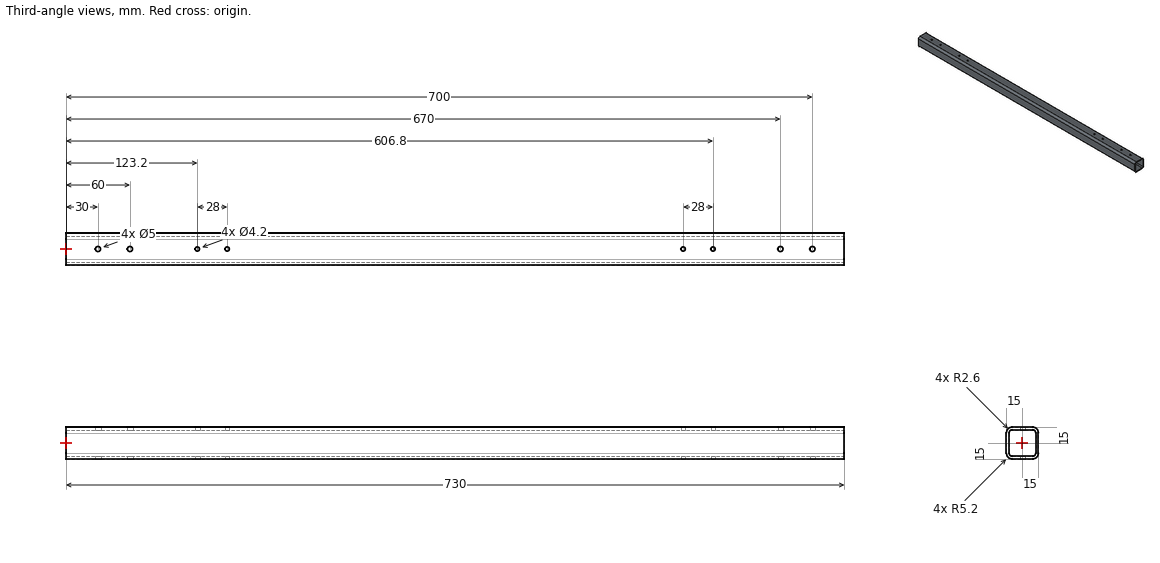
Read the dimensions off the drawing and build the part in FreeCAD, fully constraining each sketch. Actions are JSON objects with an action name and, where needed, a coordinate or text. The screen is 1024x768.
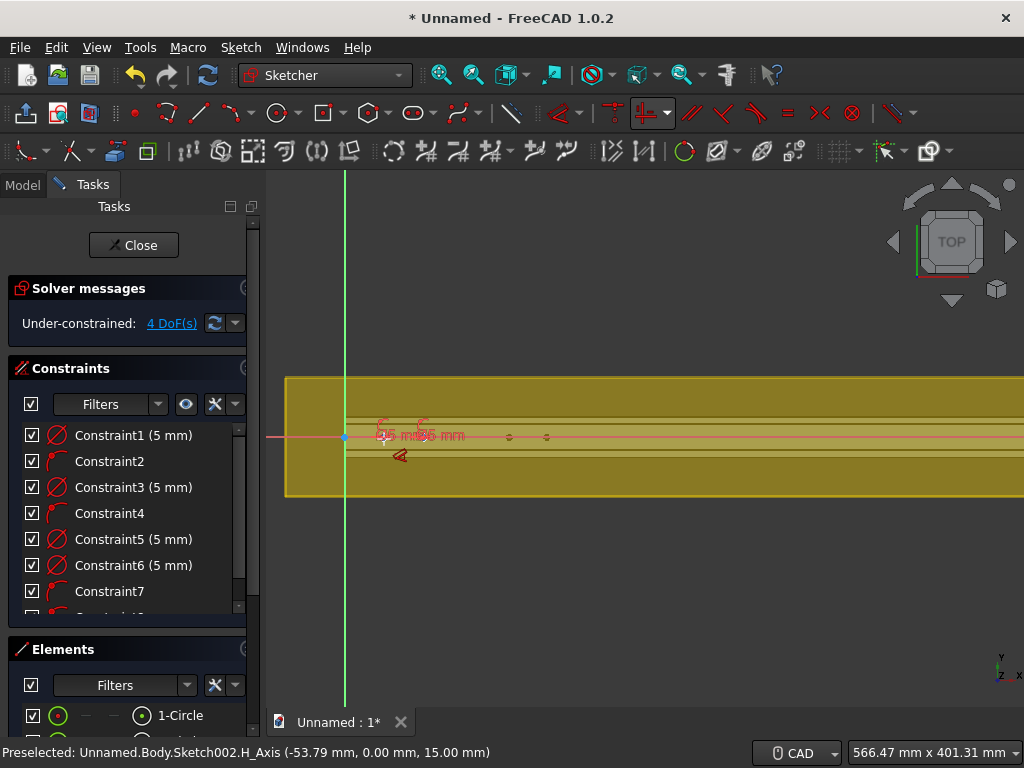
{"action": "left_click", "coordinate": [384, 437]}
{"action": "left_click", "coordinate": [364, 471]}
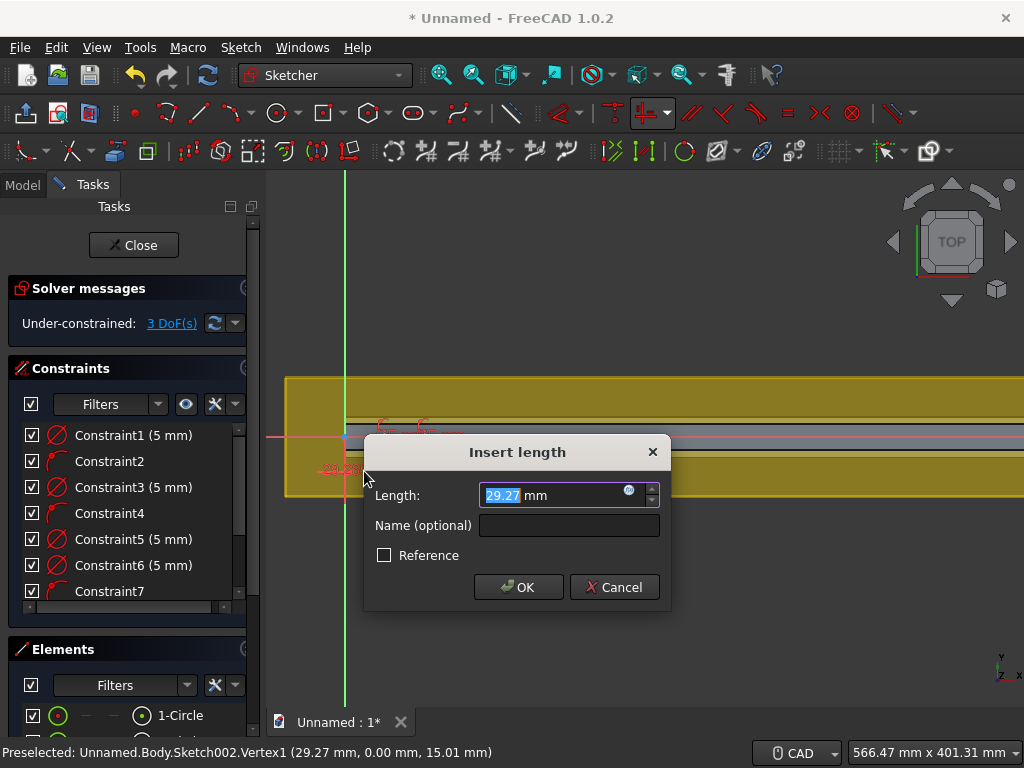
{"action": "type", "text": "30"}
{"action": "key", "text": "Return"}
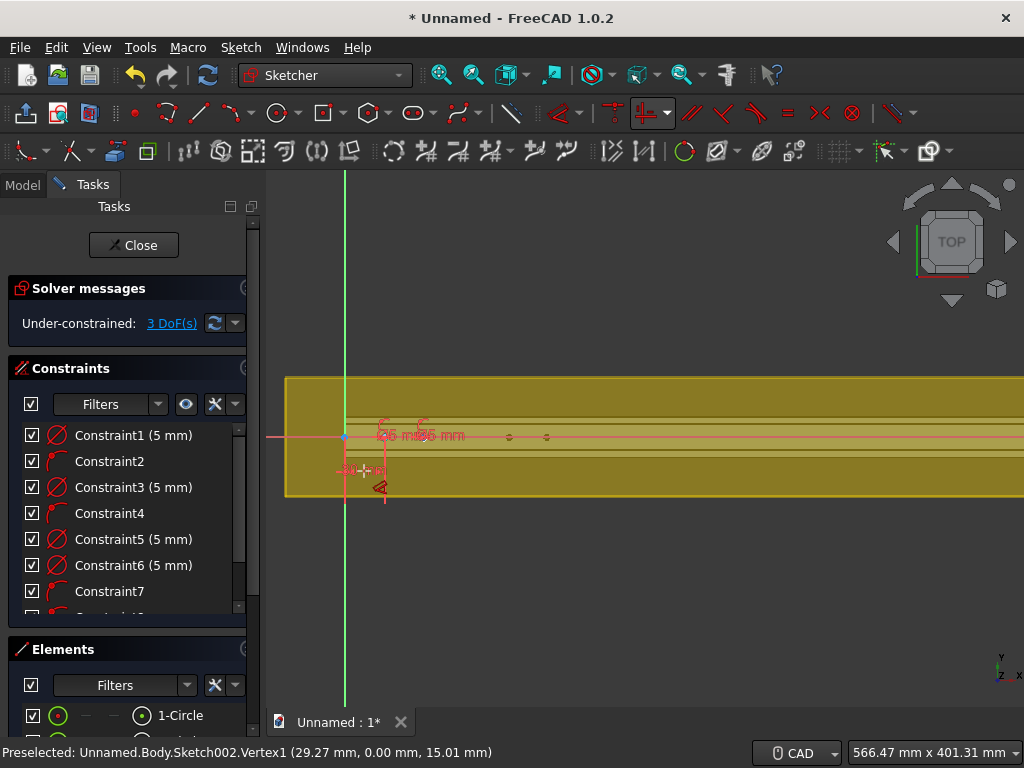
{"action": "left_click", "coordinate": [424, 437]}
{"action": "left_click", "coordinate": [384, 403]}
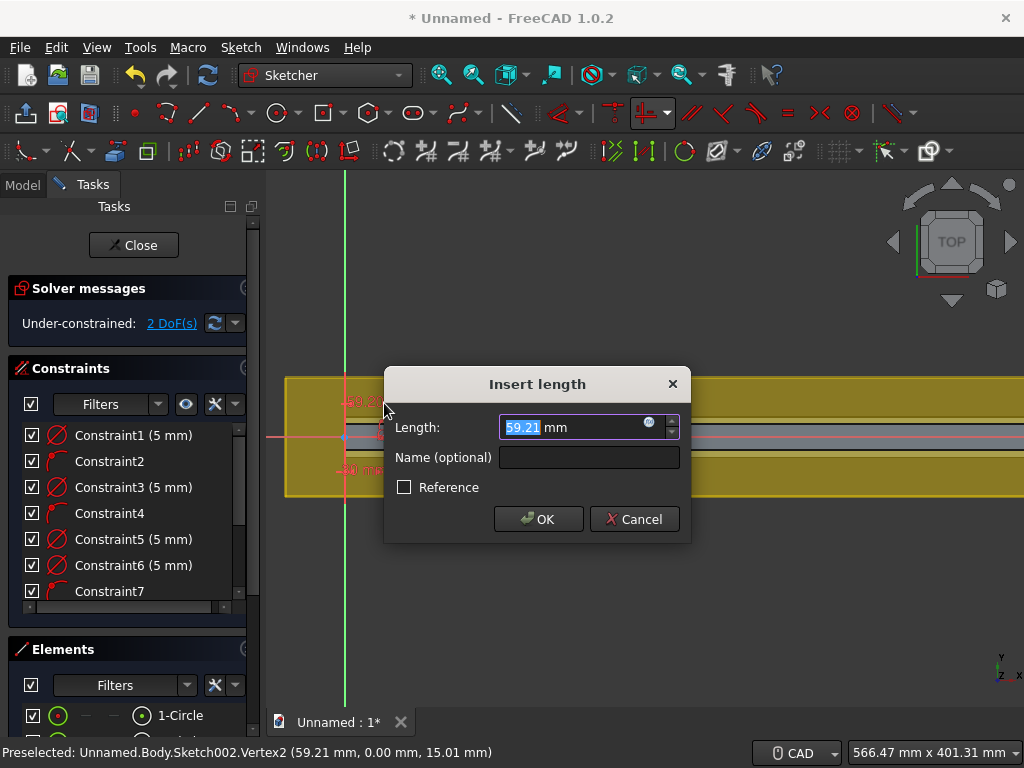
{"action": "type", "text": "60"}
{"action": "key", "text": "Return"}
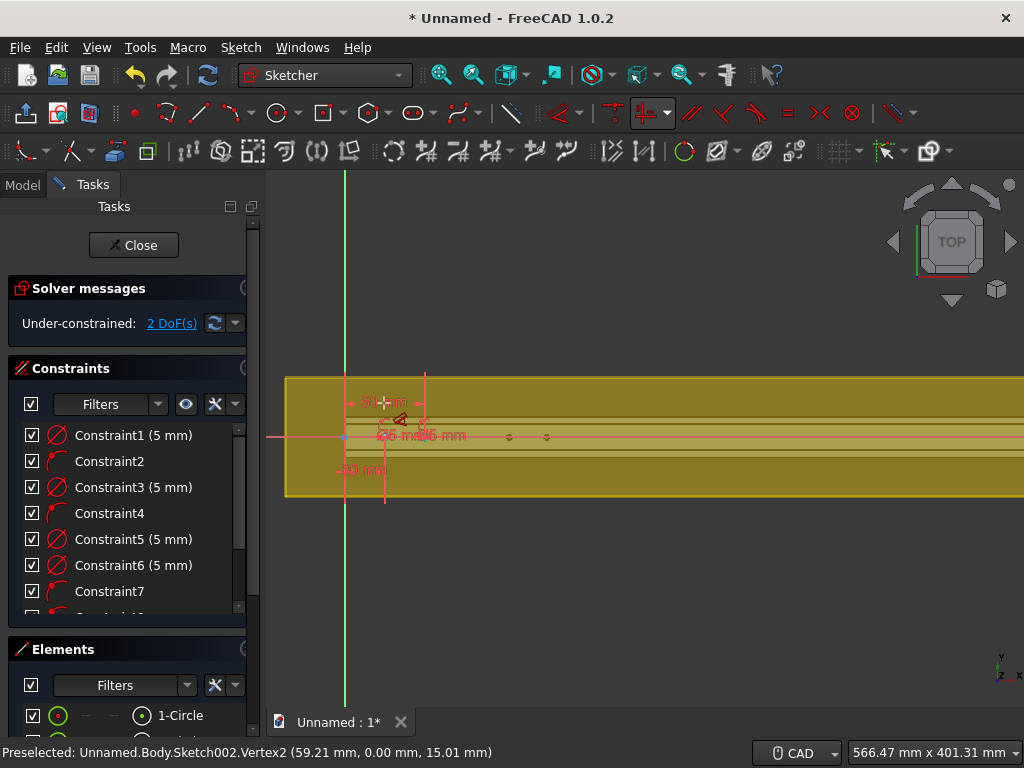
{"action": "scroll", "coordinate": [382, 439], "scroll_direction": "down", "scroll_amount": 4}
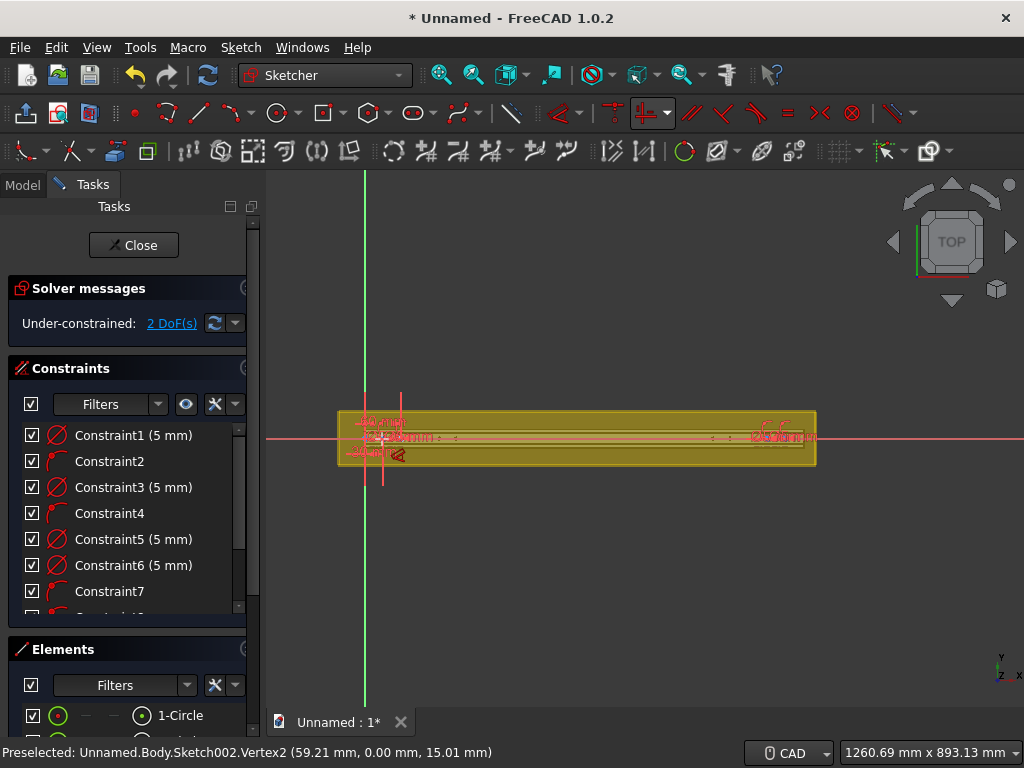
{"action": "left_click", "coordinate": [786, 439]}
{"action": "left_click", "coordinate": [576, 473]}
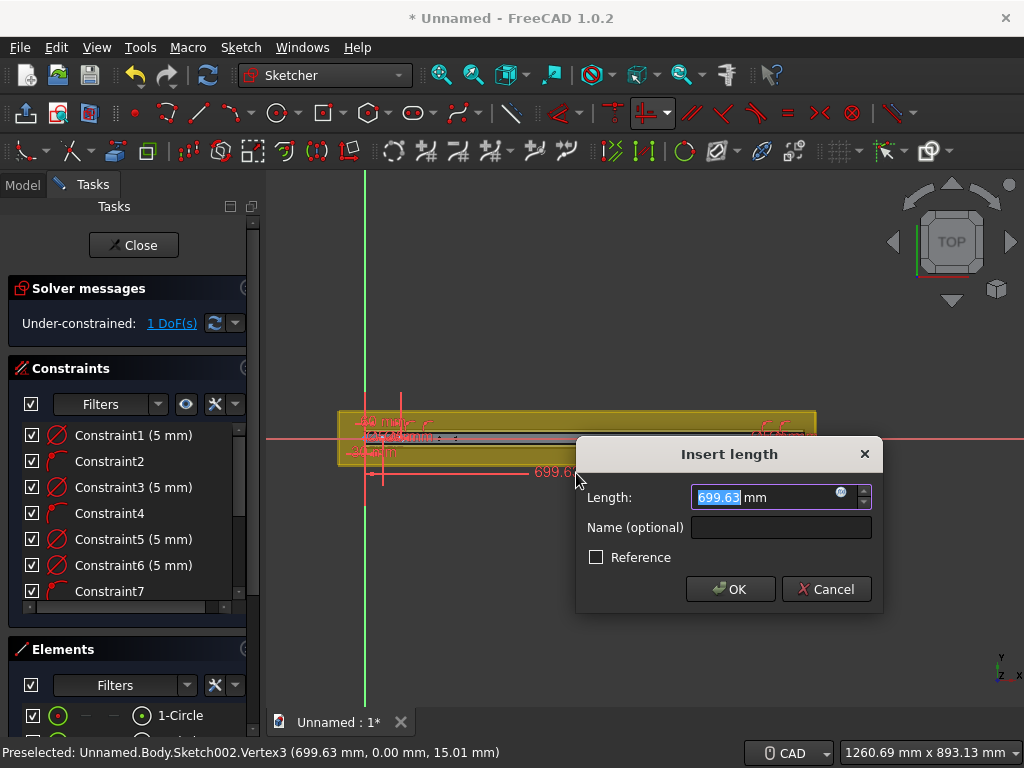
{"action": "type", "text": "700"}
{"action": "key", "text": "Return"}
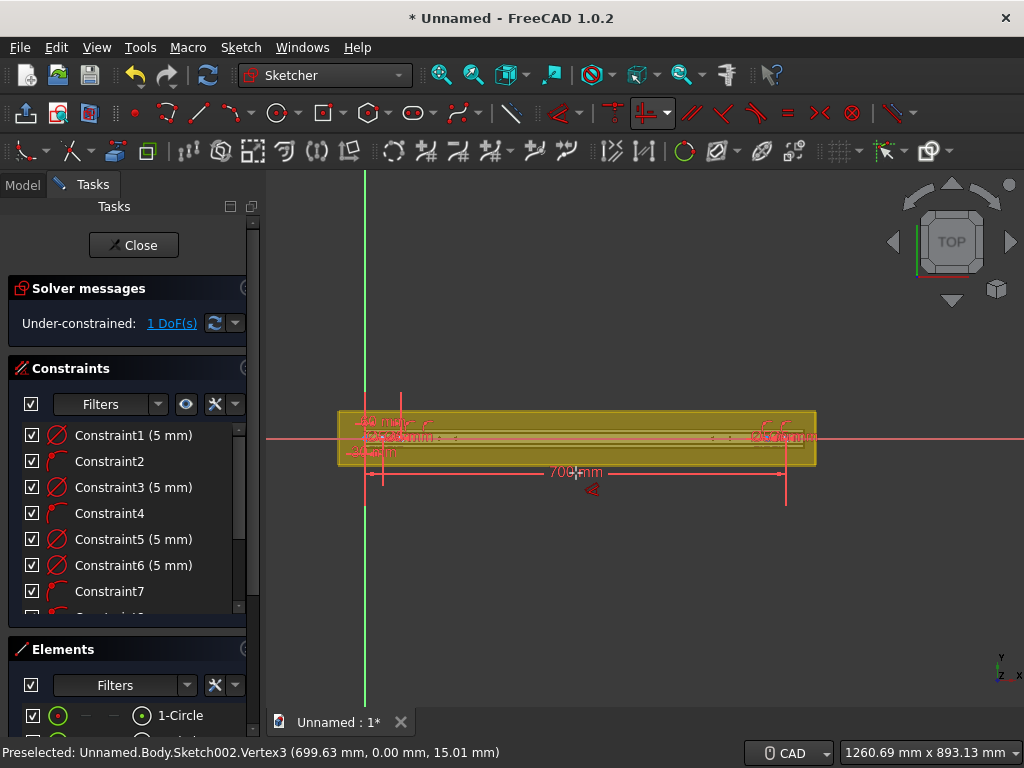
{"action": "left_click", "coordinate": [768, 439]}
{"action": "left_click", "coordinate": [474, 473]}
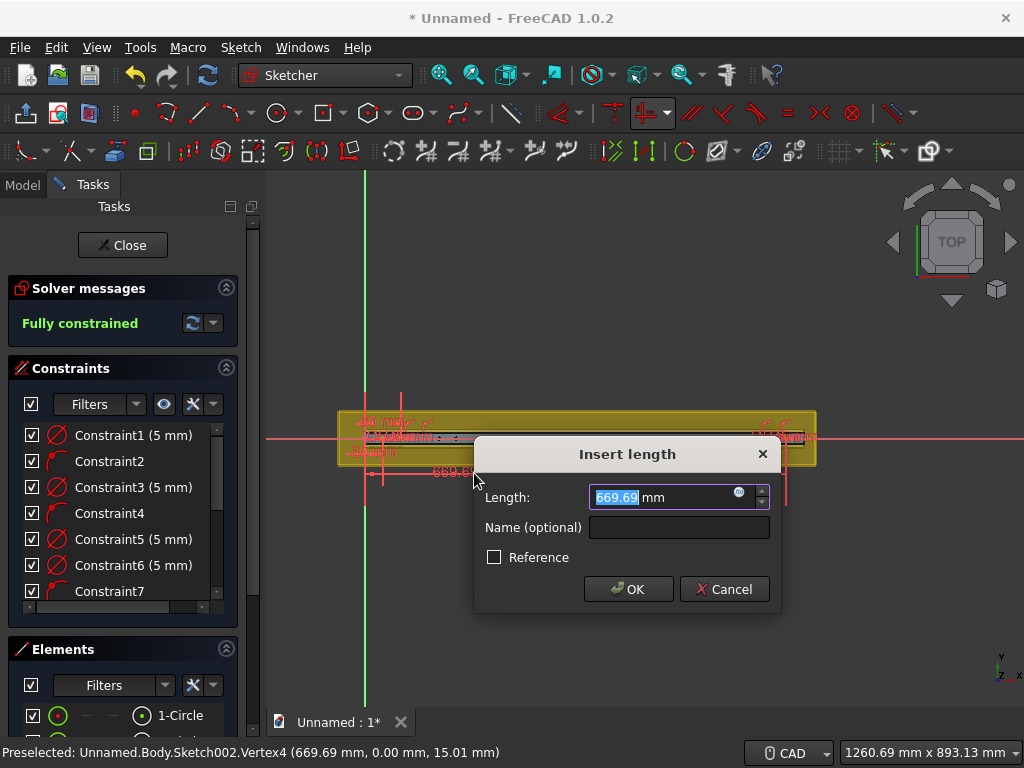
{"action": "type", "text": "670"}
{"action": "key", "text": "Return"}
{"action": "key", "text": "Escape"}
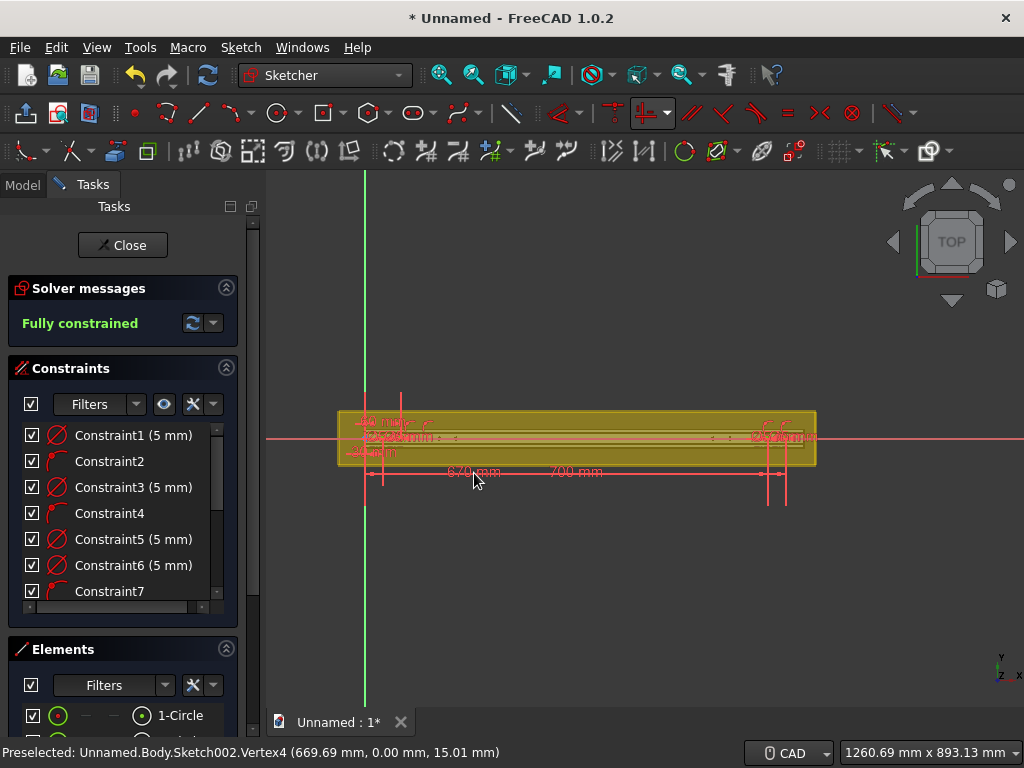
{"action": "left_click", "coordinate": [123, 245]}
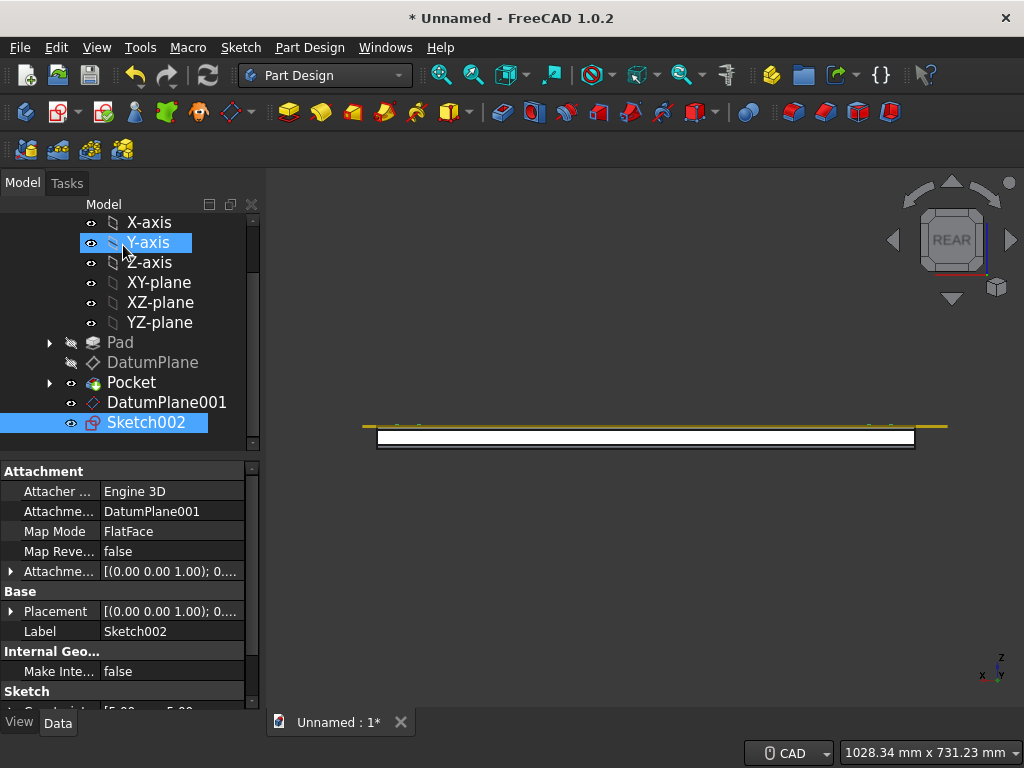
{"action": "left_click", "coordinate": [504, 112]}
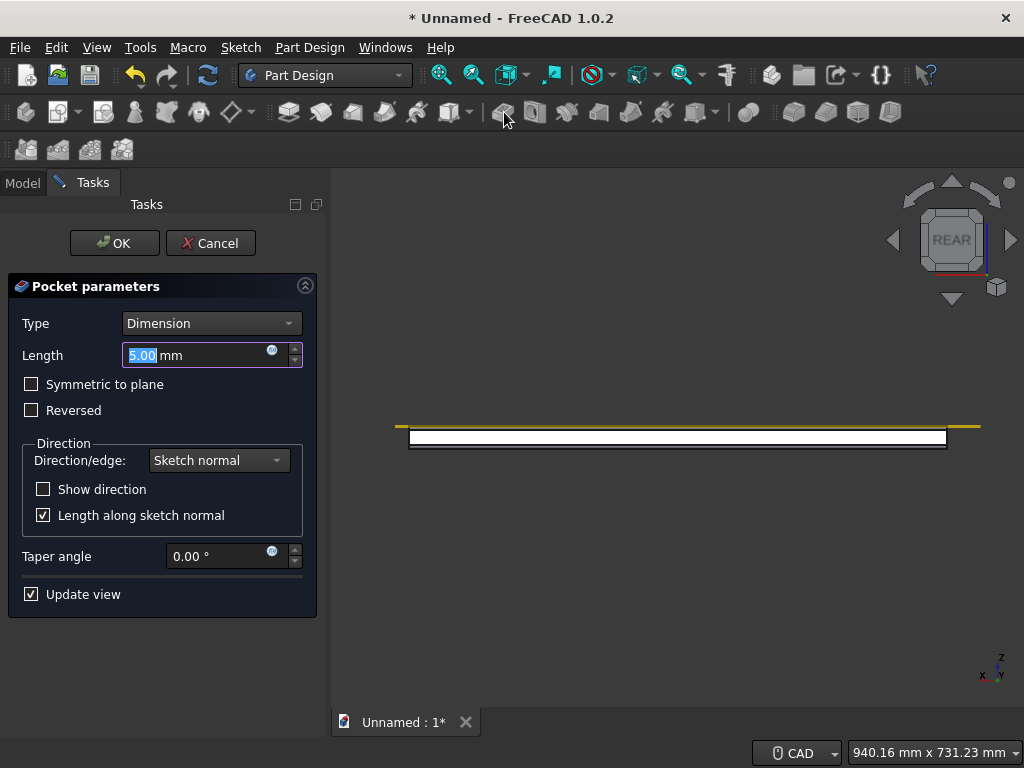
{"action": "left_click", "coordinate": [212, 324]}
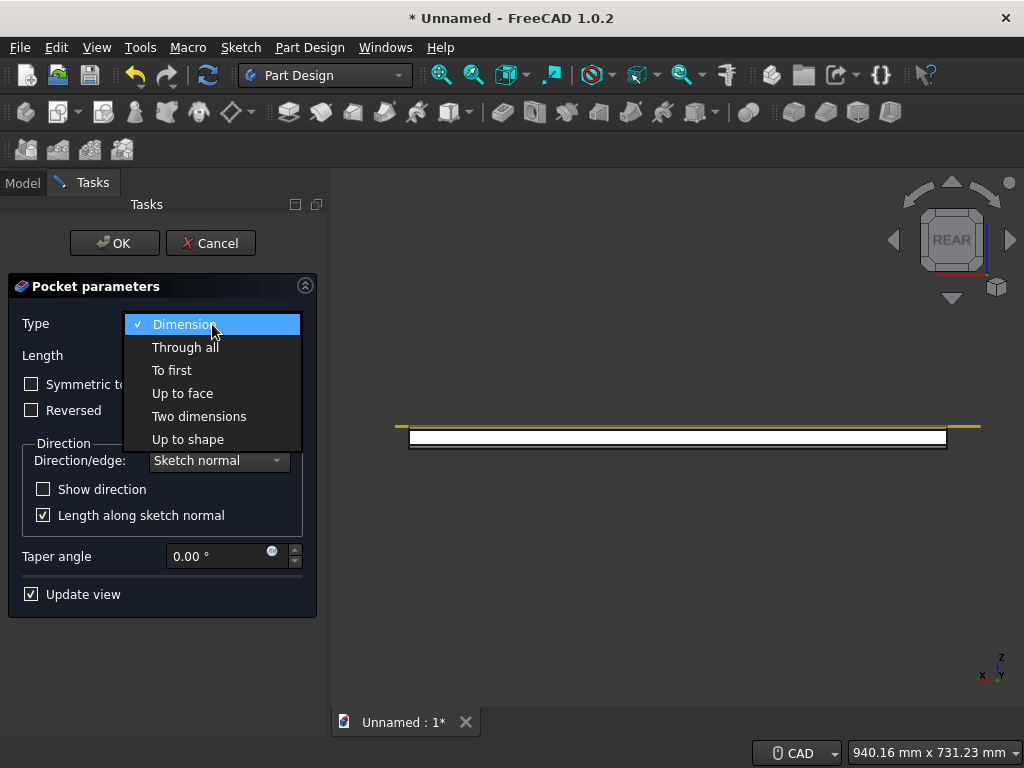
{"action": "left_click", "coordinate": [212, 348]}